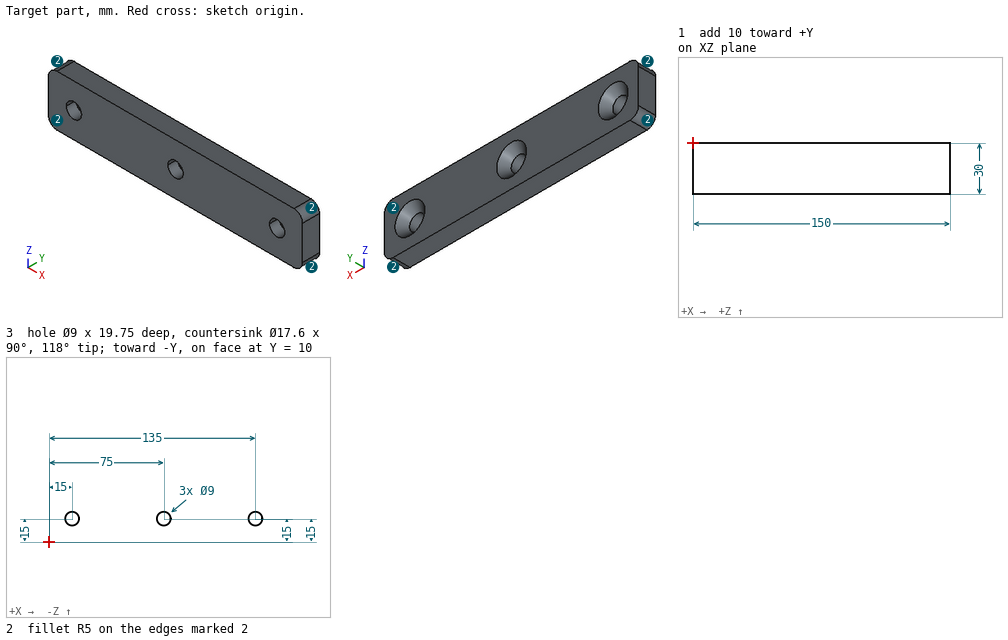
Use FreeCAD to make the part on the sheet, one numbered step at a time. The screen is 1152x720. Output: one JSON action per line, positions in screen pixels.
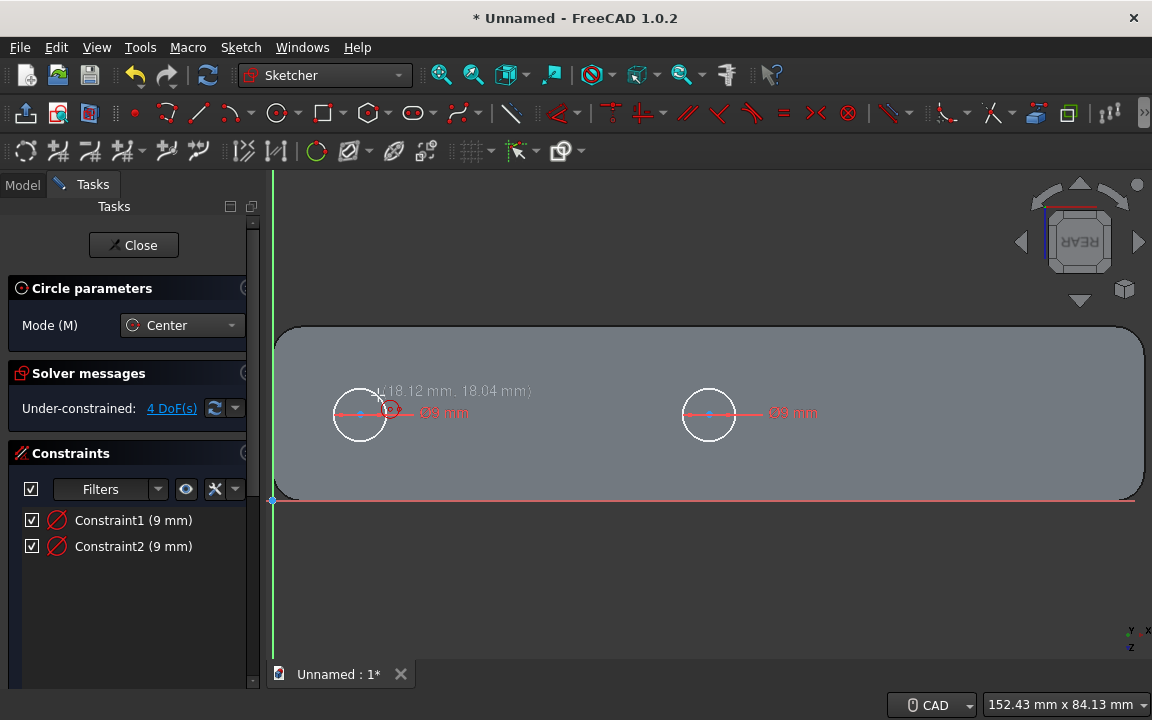
{"action": "scroll", "coordinate": [595, 378], "scroll_direction": "down", "scroll_amount": 3}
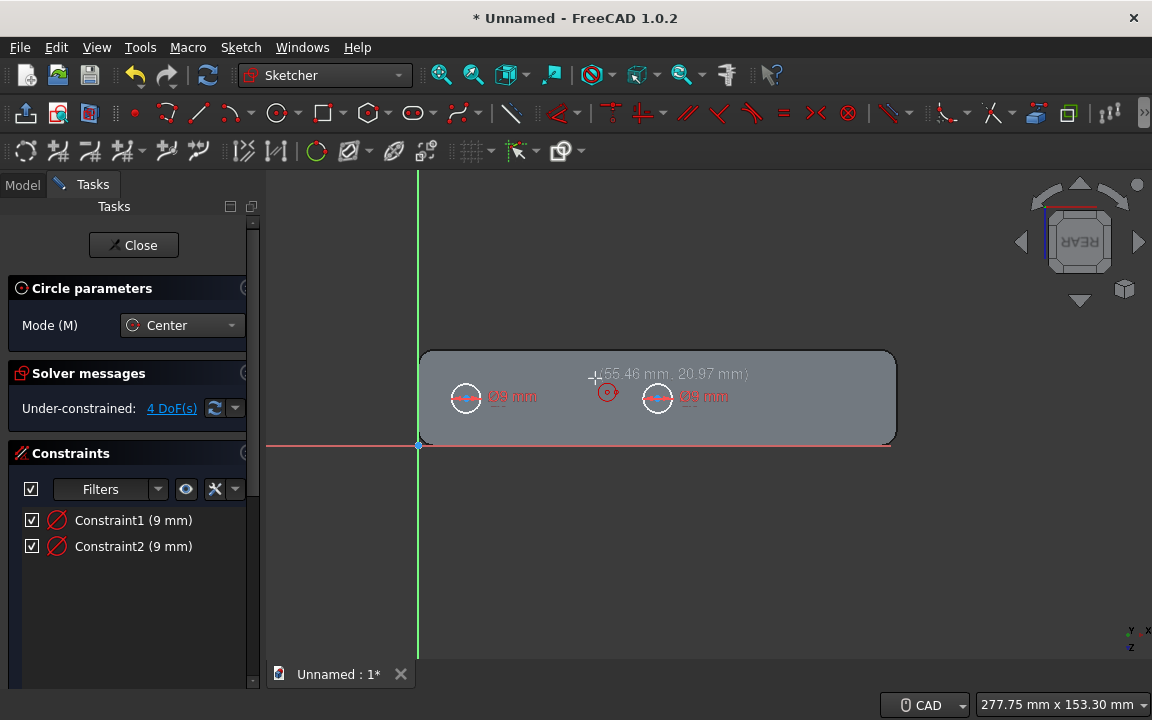
{"action": "scroll", "coordinate": [849, 398], "scroll_direction": "up", "scroll_amount": 3}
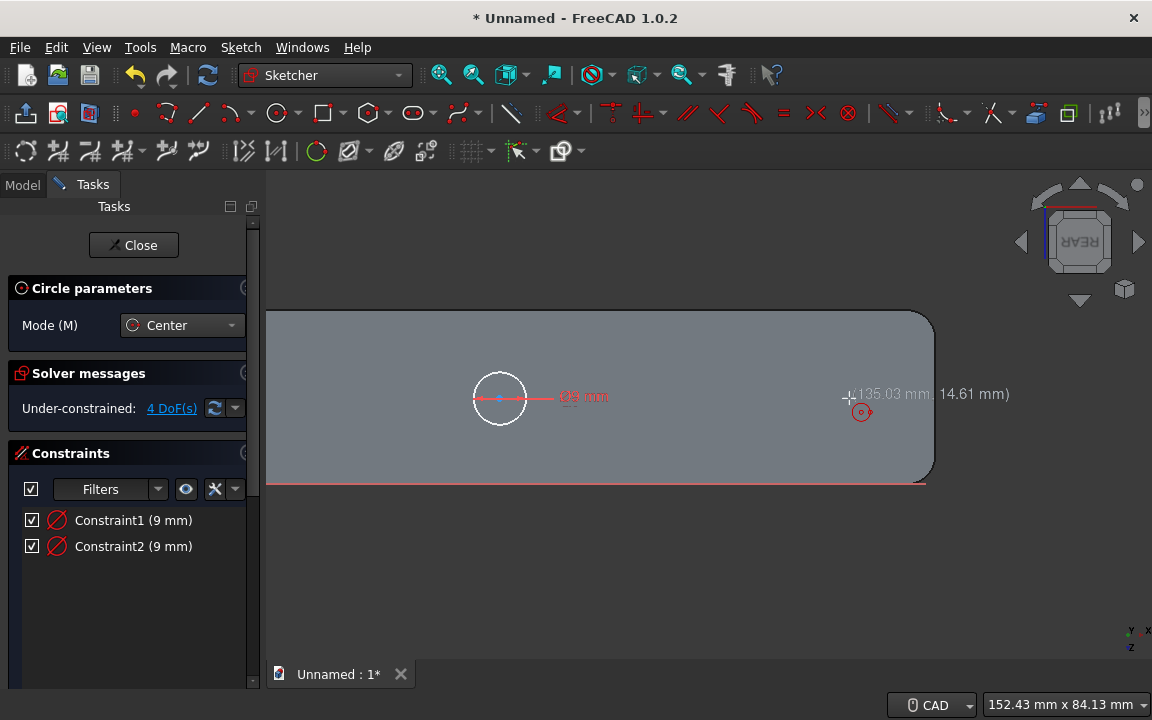
{"action": "left_click", "coordinate": [848, 397]}
{"action": "mouse_move", "coordinate": [867, 379]}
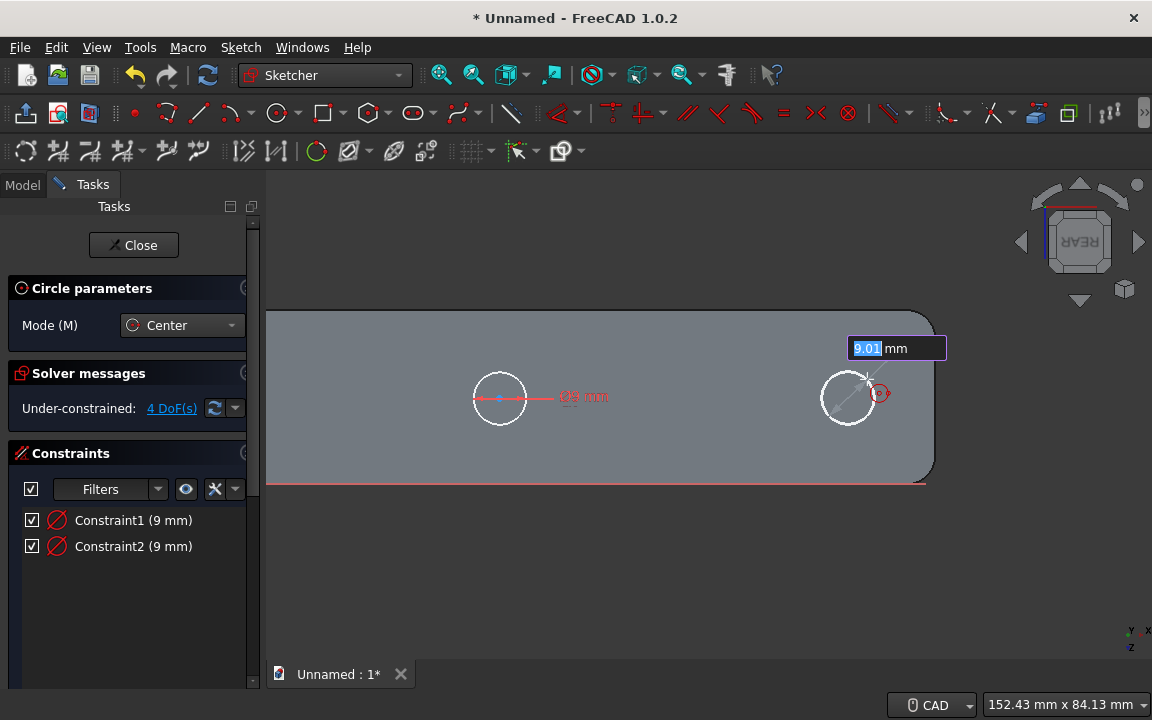
{"action": "type", "text": "9"}
{"action": "key", "text": "Return"}
{"action": "key", "text": "Escape"}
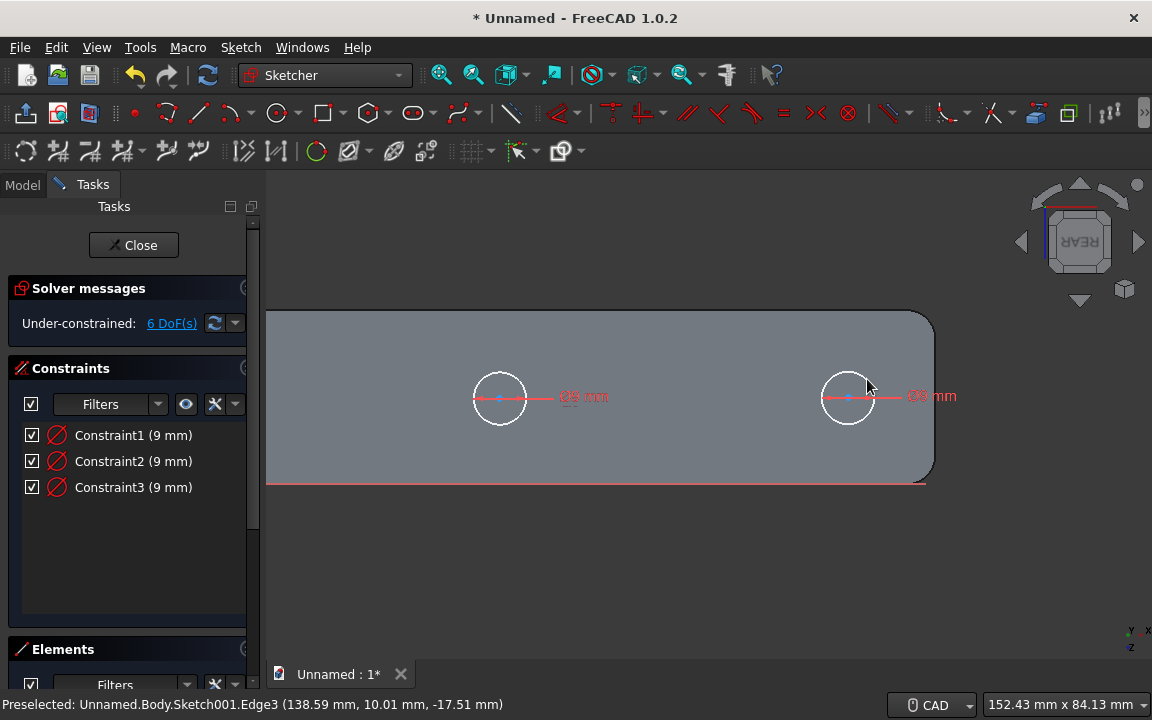
{"action": "left_click", "coordinate": [558, 114]}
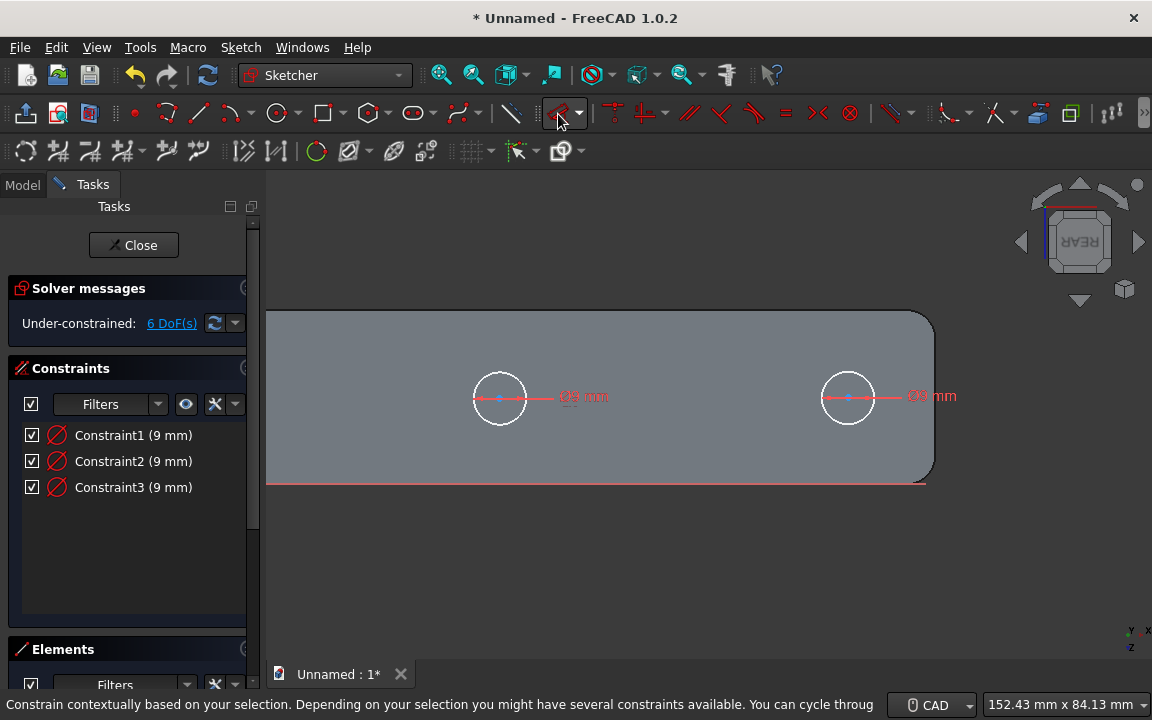
{"action": "left_click", "coordinate": [500, 399]}
{"action": "left_click", "coordinate": [397, 518]}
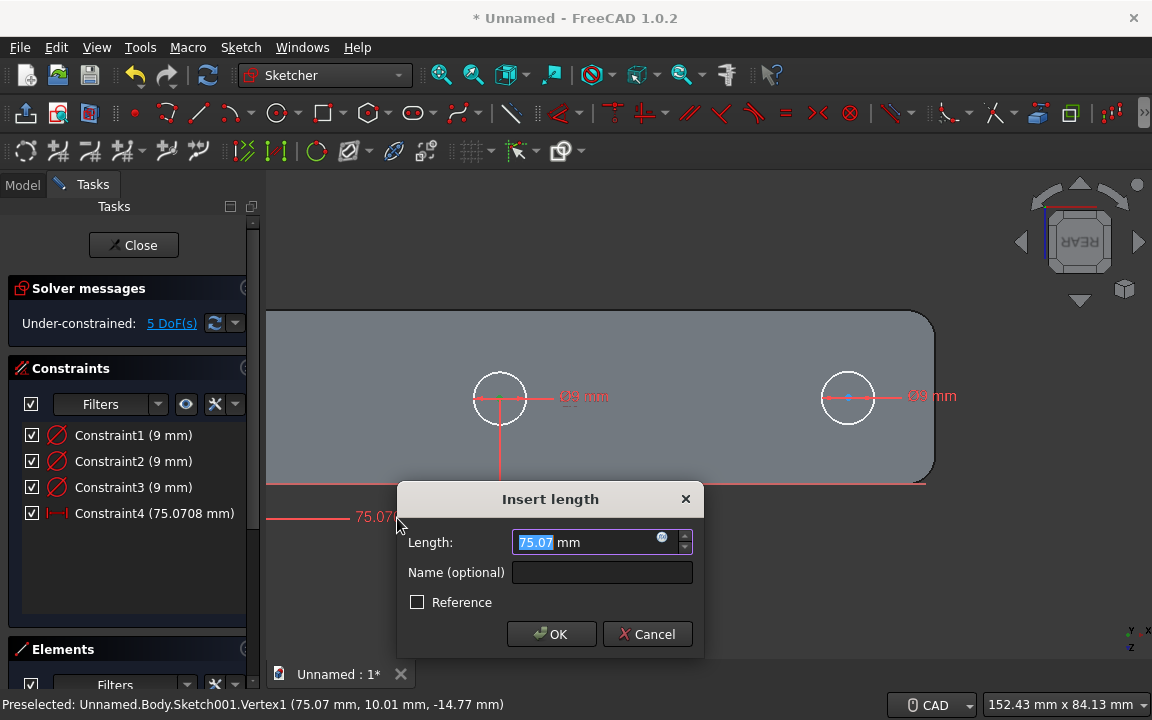
{"action": "type", "text": "75"}
{"action": "key", "text": "Return"}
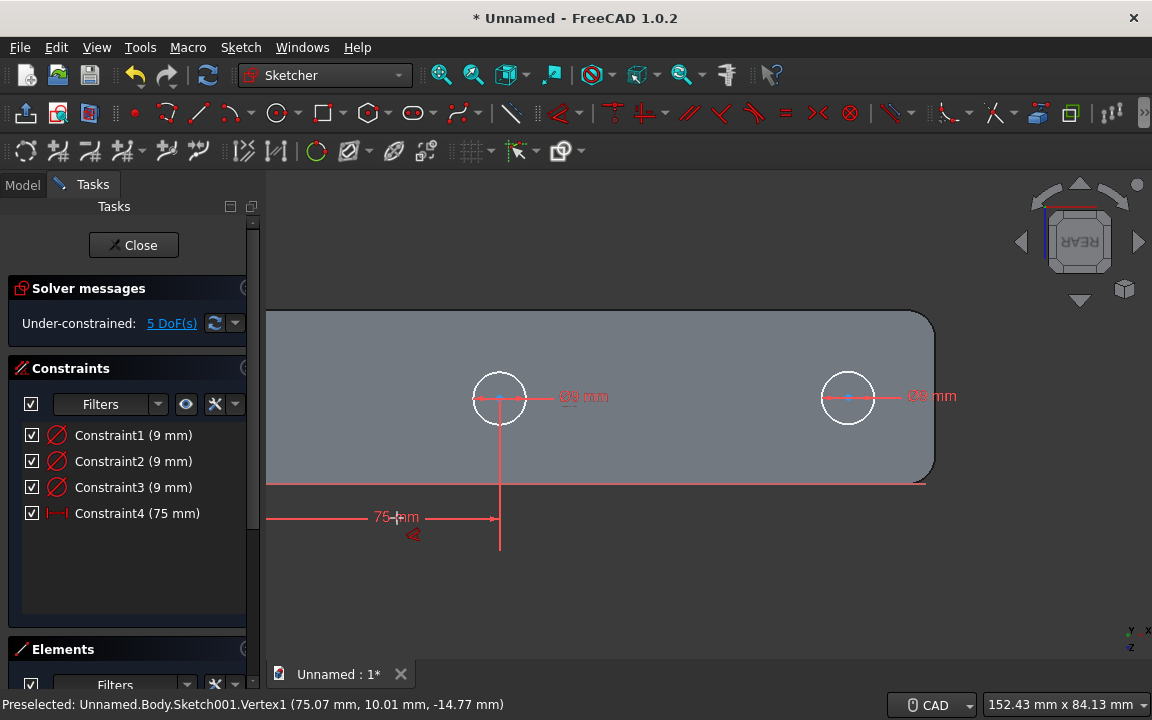
{"action": "left_click", "coordinate": [500, 399]}
{"action": "left_click", "coordinate": [534, 441]}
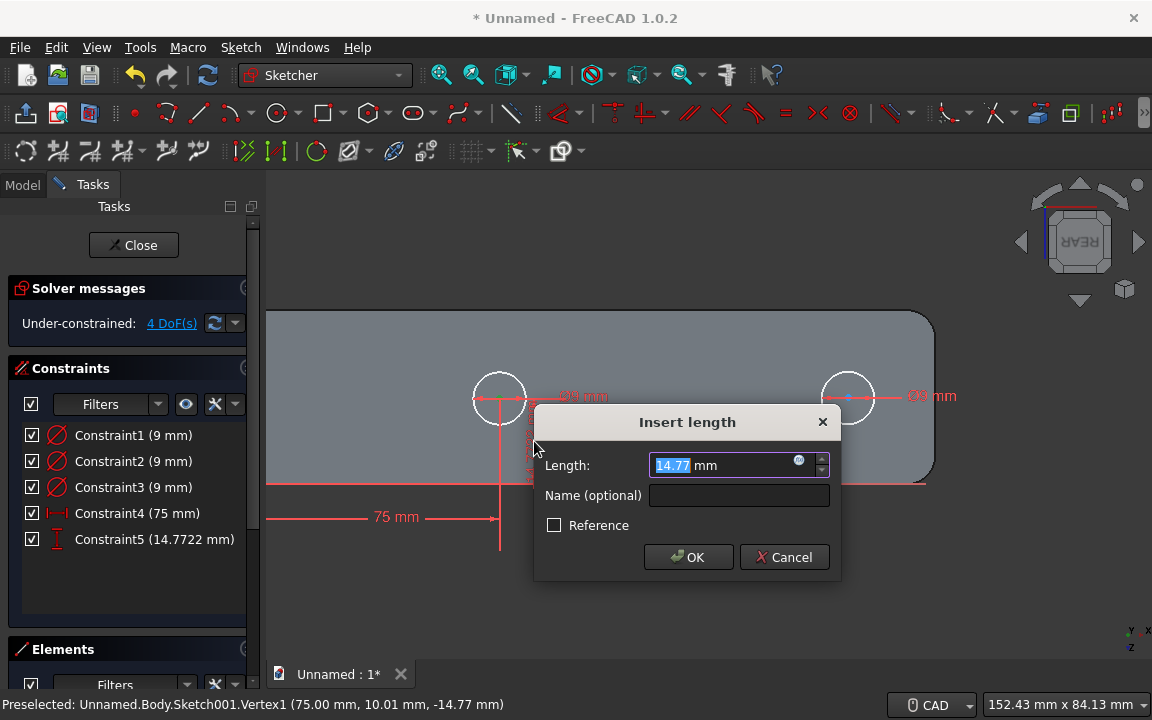
{"action": "type", "text": "15"}
{"action": "key", "text": "Return"}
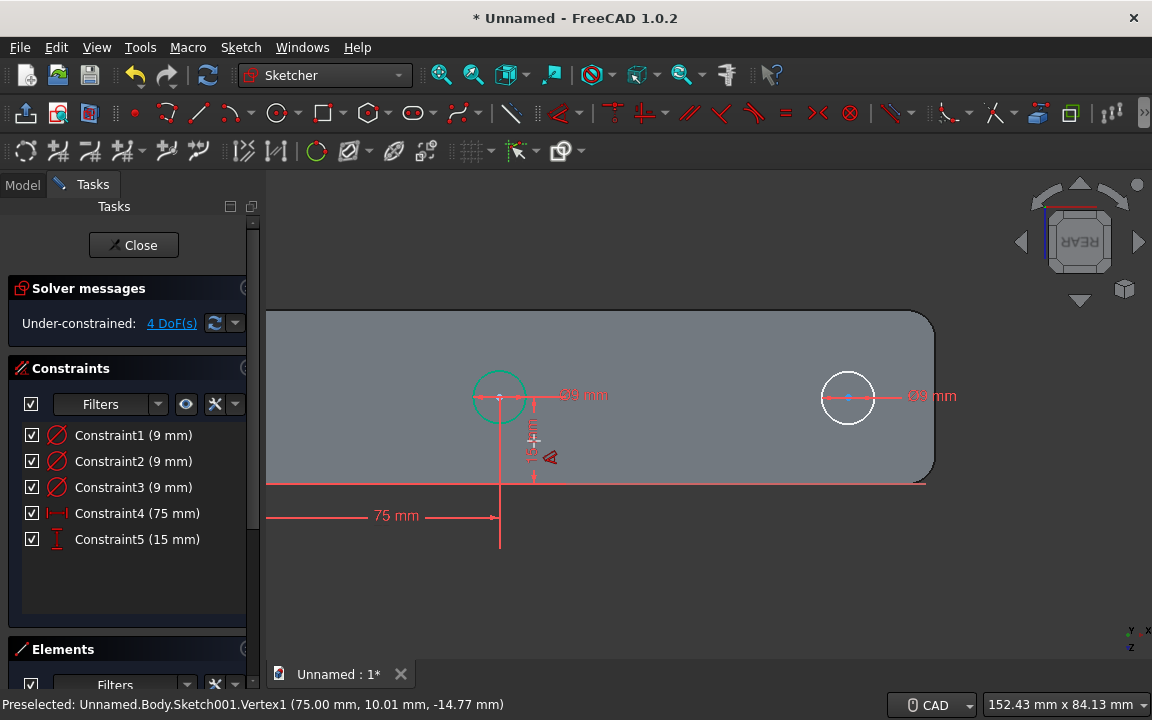
{"action": "scroll", "coordinate": [849, 398], "scroll_direction": "down", "scroll_amount": 3}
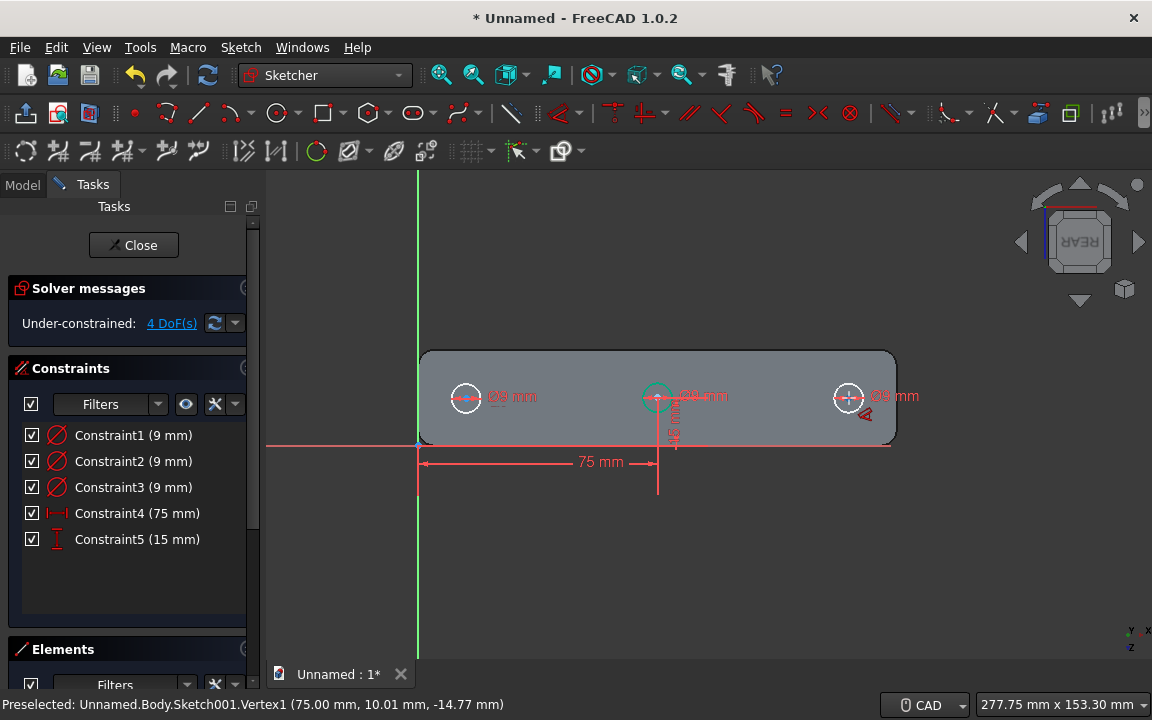
{"action": "left_click", "coordinate": [466, 398]}
{"action": "left_click", "coordinate": [442, 480]}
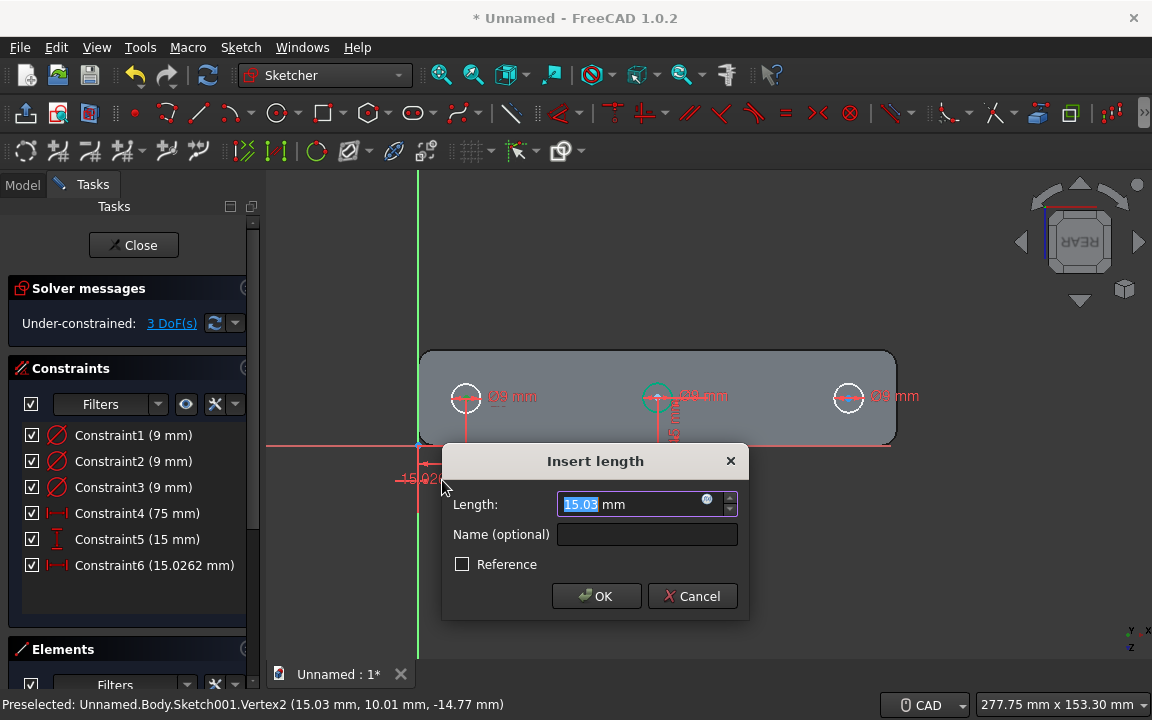
{"action": "type", "text": "15"}
{"action": "key", "text": "Return"}